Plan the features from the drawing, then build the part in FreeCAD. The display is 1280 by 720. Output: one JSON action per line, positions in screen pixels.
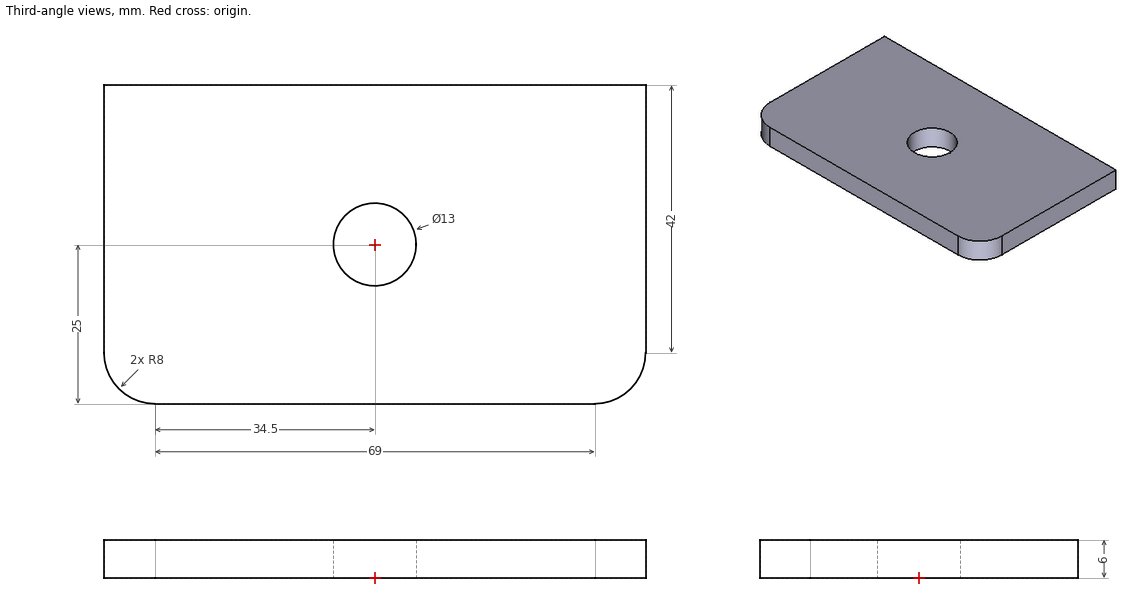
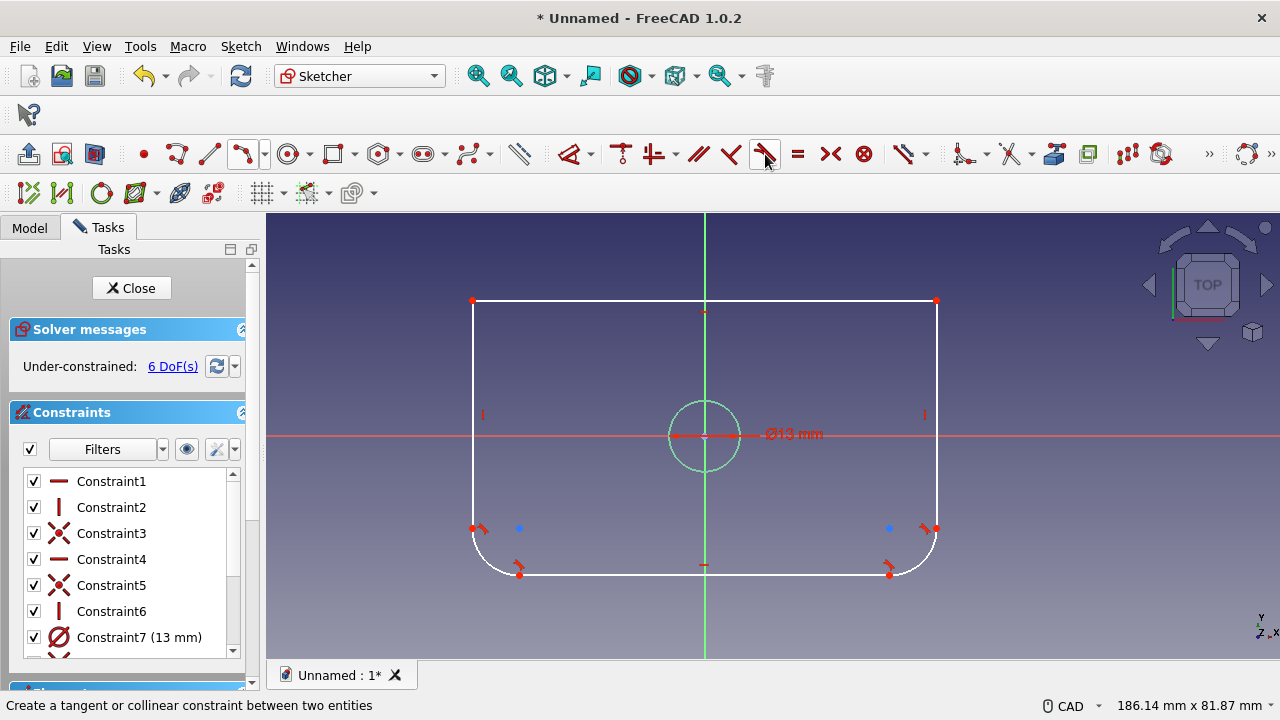
{"action": "left_click", "coordinate": [911, 570]}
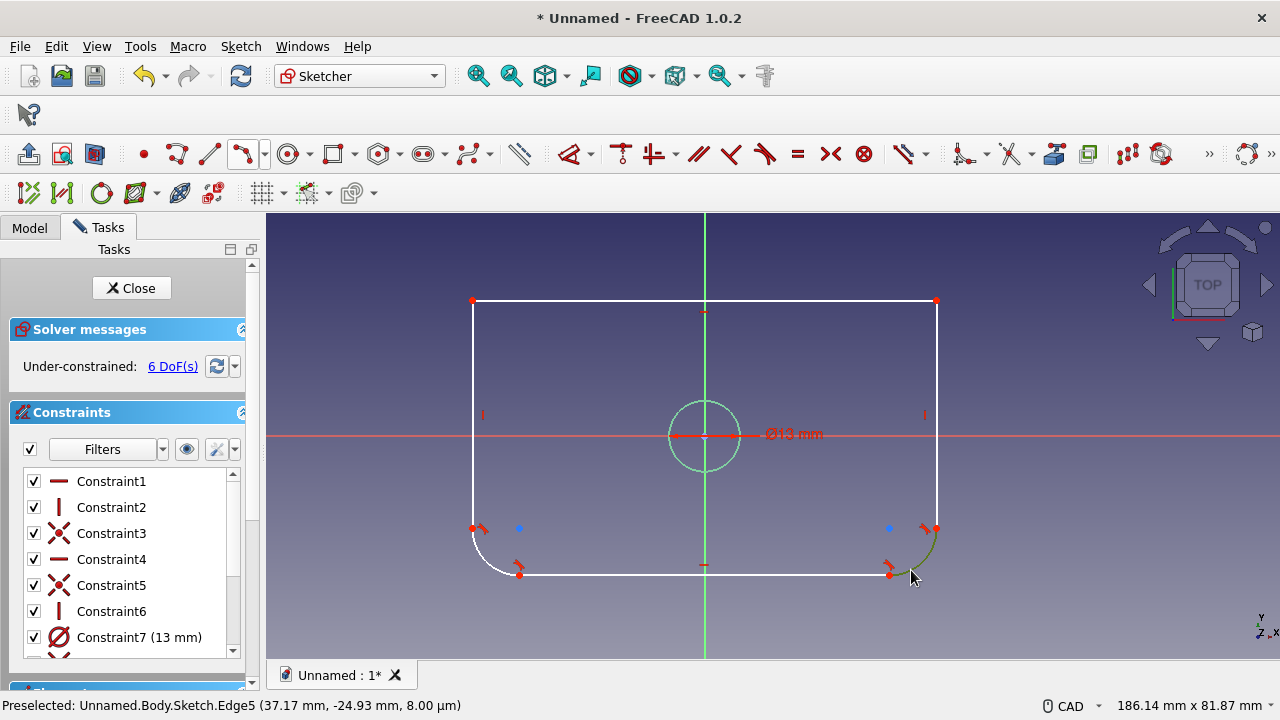
{"action": "left_click", "coordinate": [478, 550]}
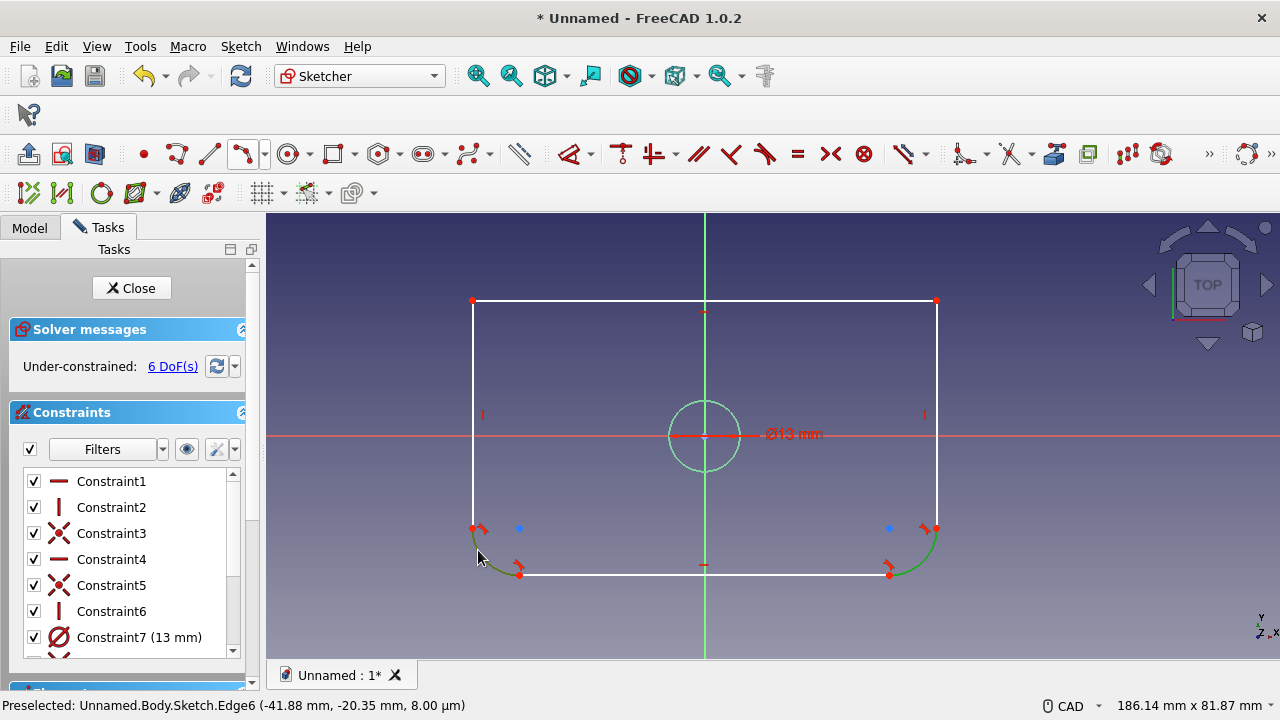
{"action": "left_click", "coordinate": [798, 154]}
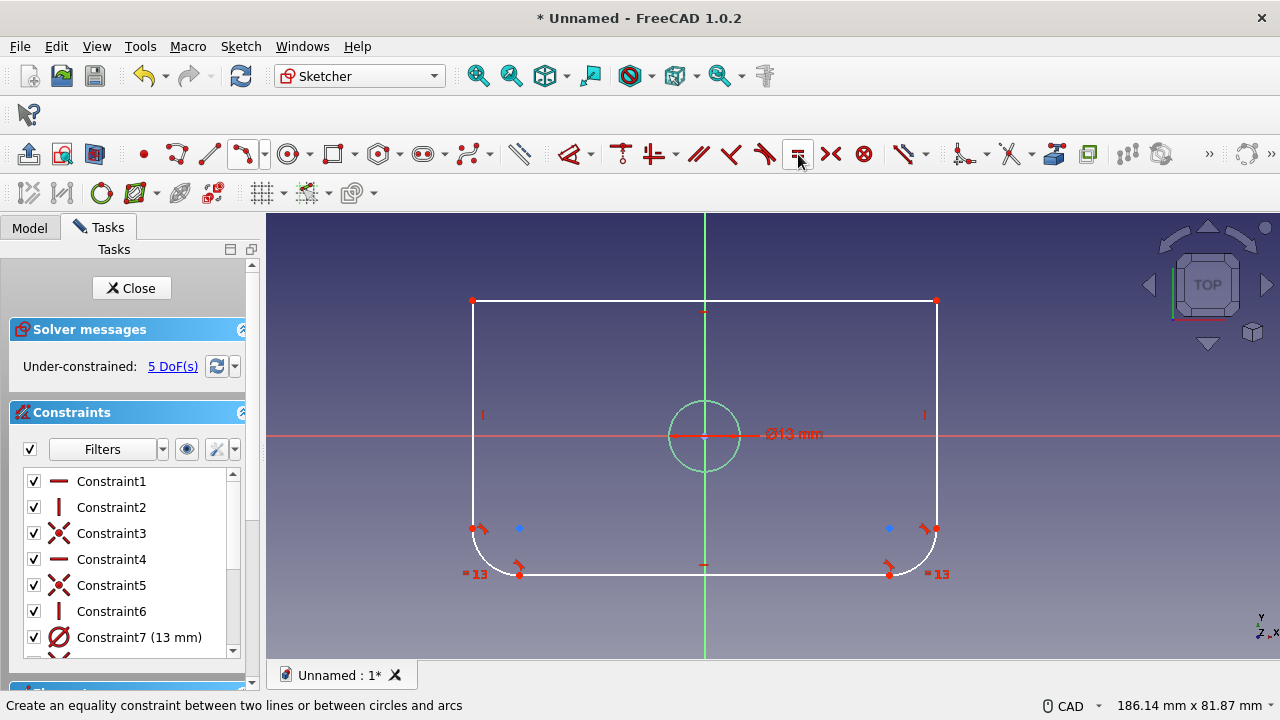
{"action": "left_click", "coordinate": [568, 154]}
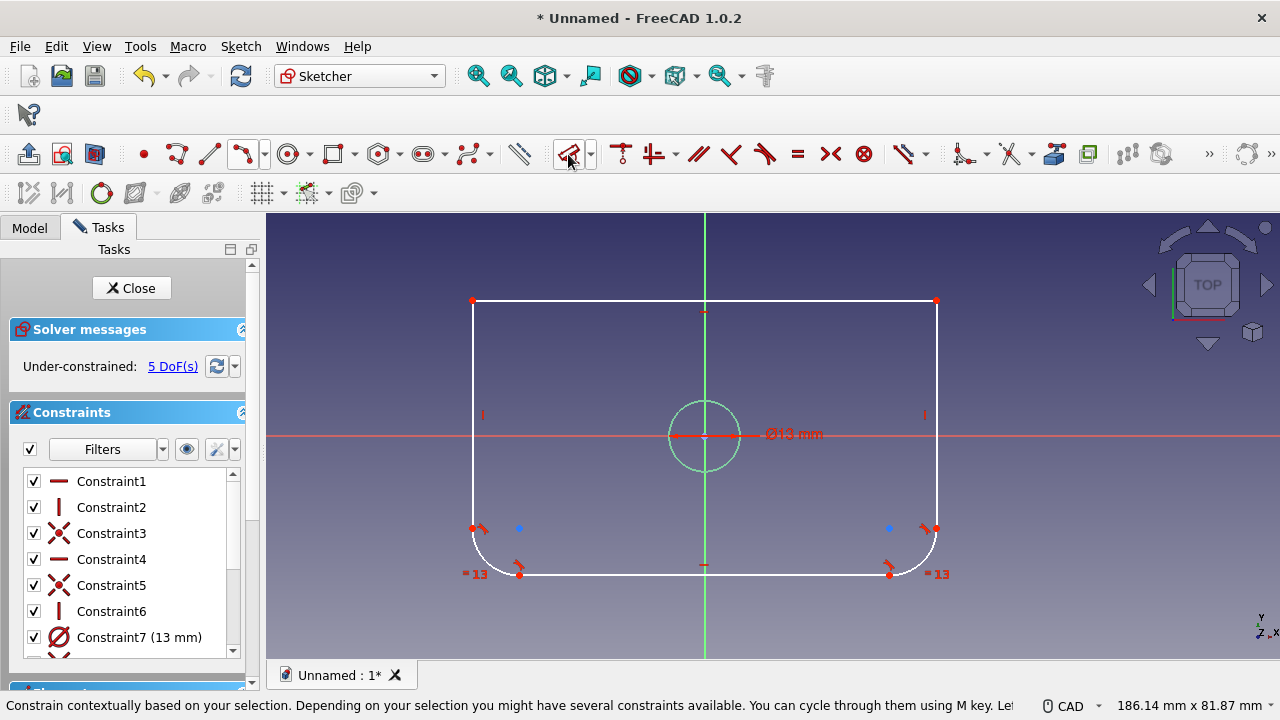
{"action": "left_click", "coordinate": [911, 570]}
{"action": "left_click", "coordinate": [926, 598]}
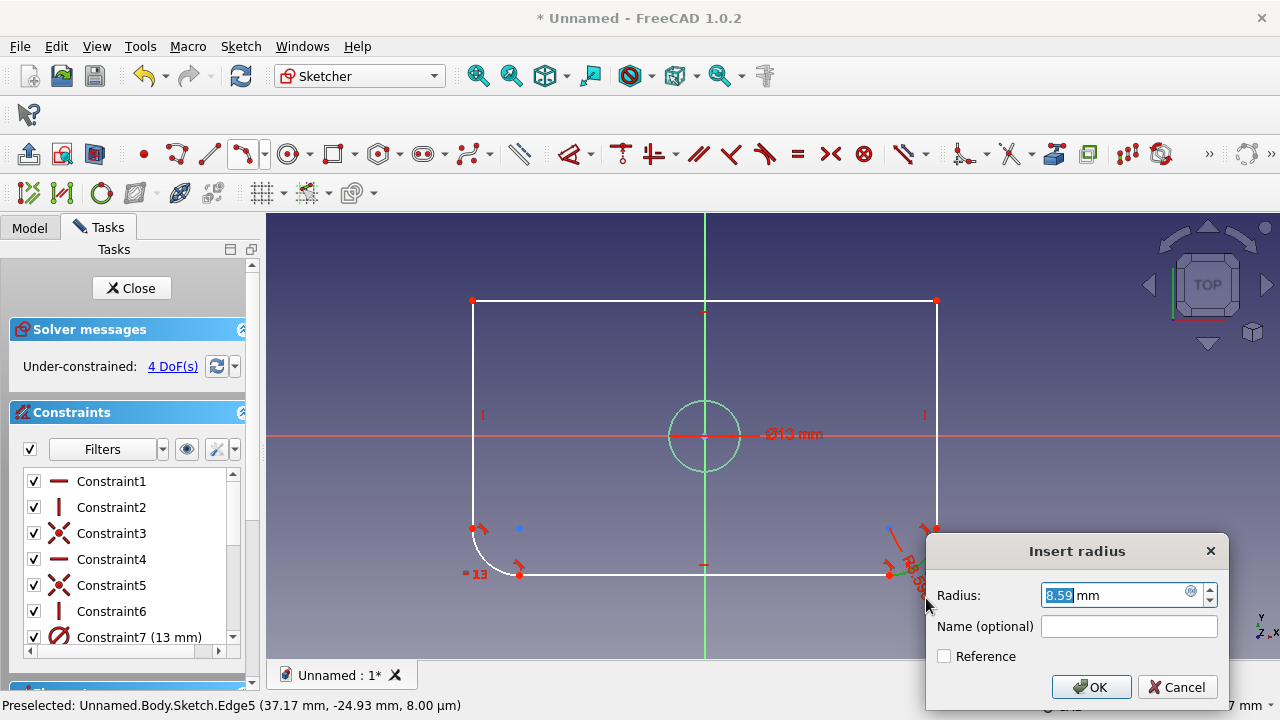
{"action": "type", "text": "8"}
{"action": "key", "text": "Return"}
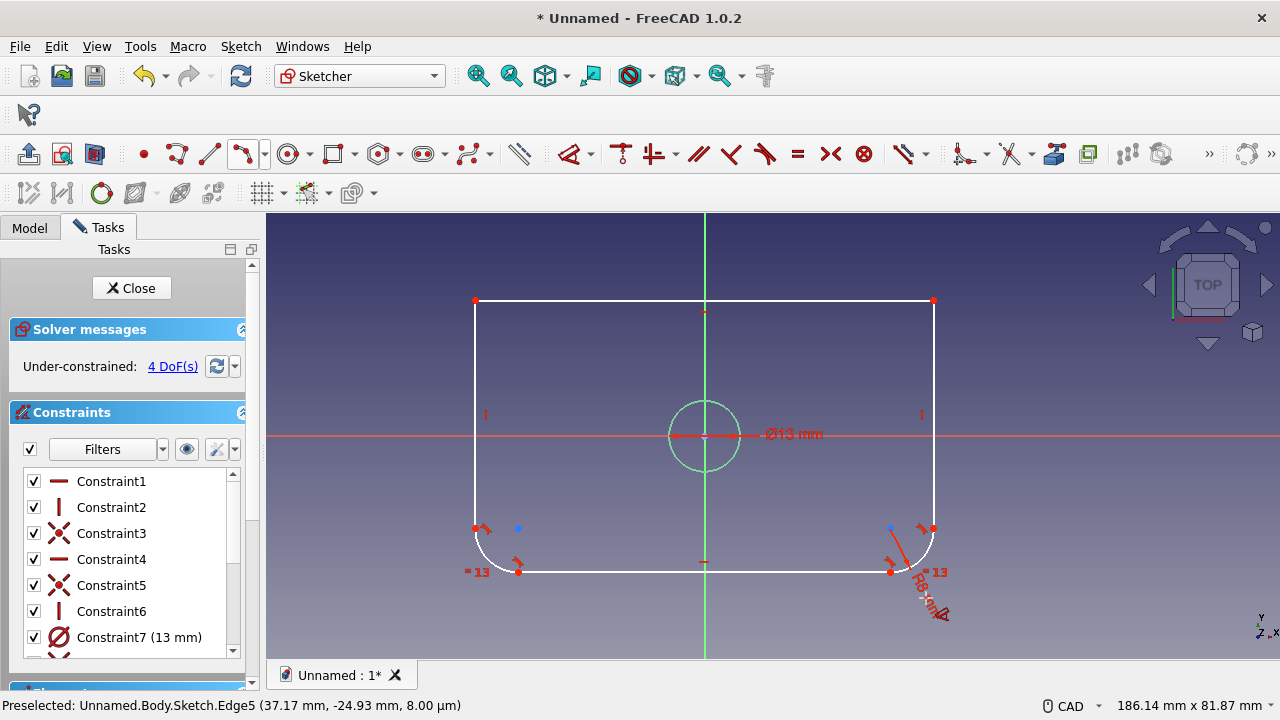
{"action": "left_click", "coordinate": [630, 572]}
{"action": "left_click", "coordinate": [619, 606]}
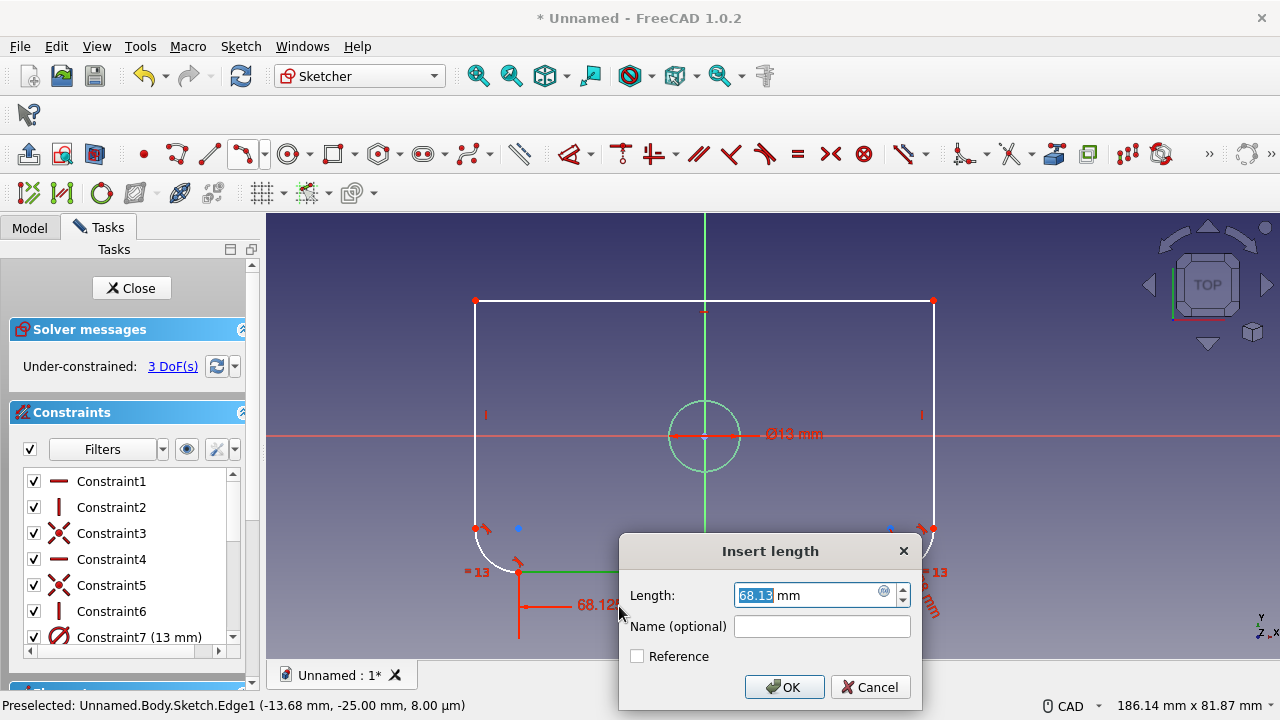
{"action": "type", "text": "69"}
{"action": "key", "text": "Return"}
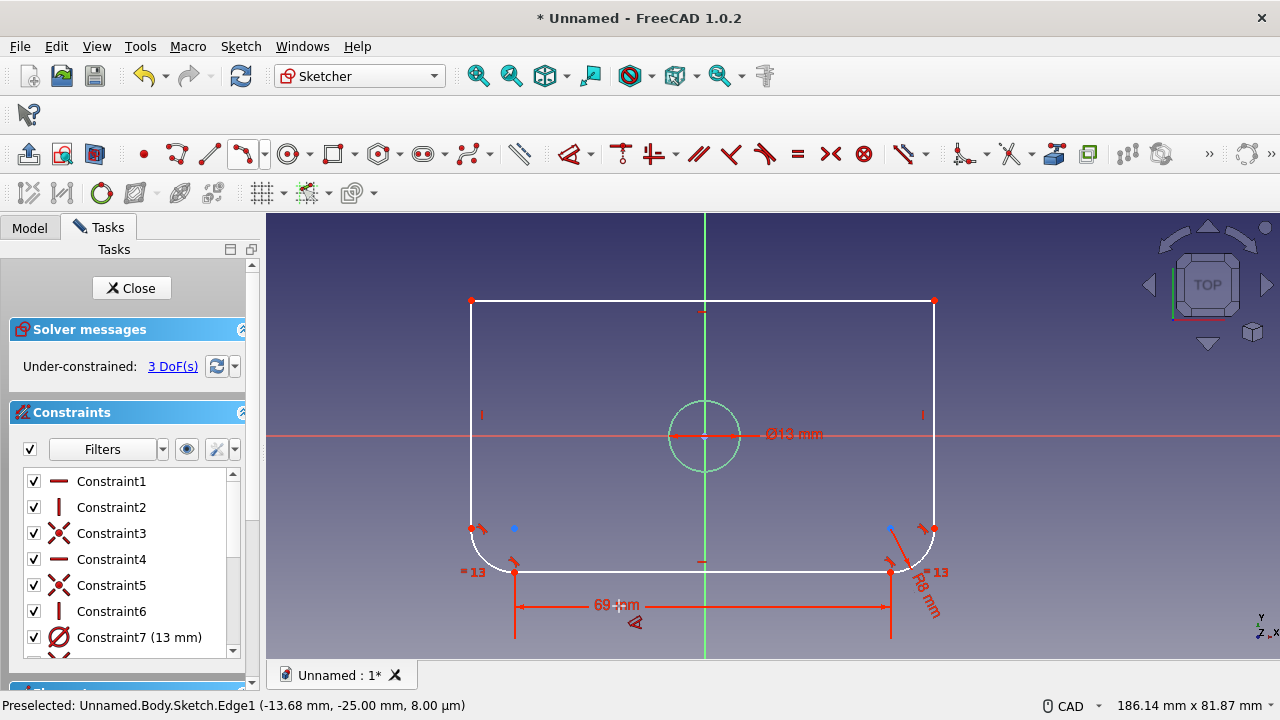
{"action": "left_click", "coordinate": [934, 460]}
{"action": "left_click", "coordinate": [968, 415]}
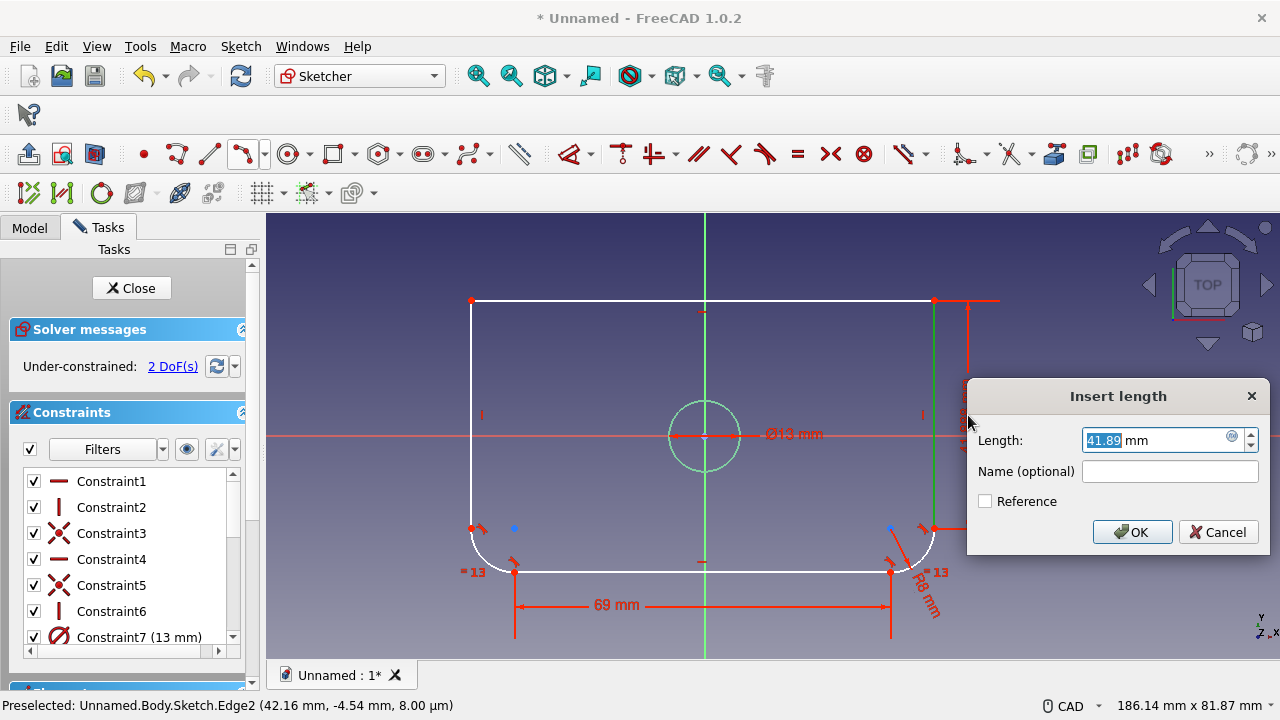
{"action": "type", "text": "42"}
{"action": "key", "text": "Return"}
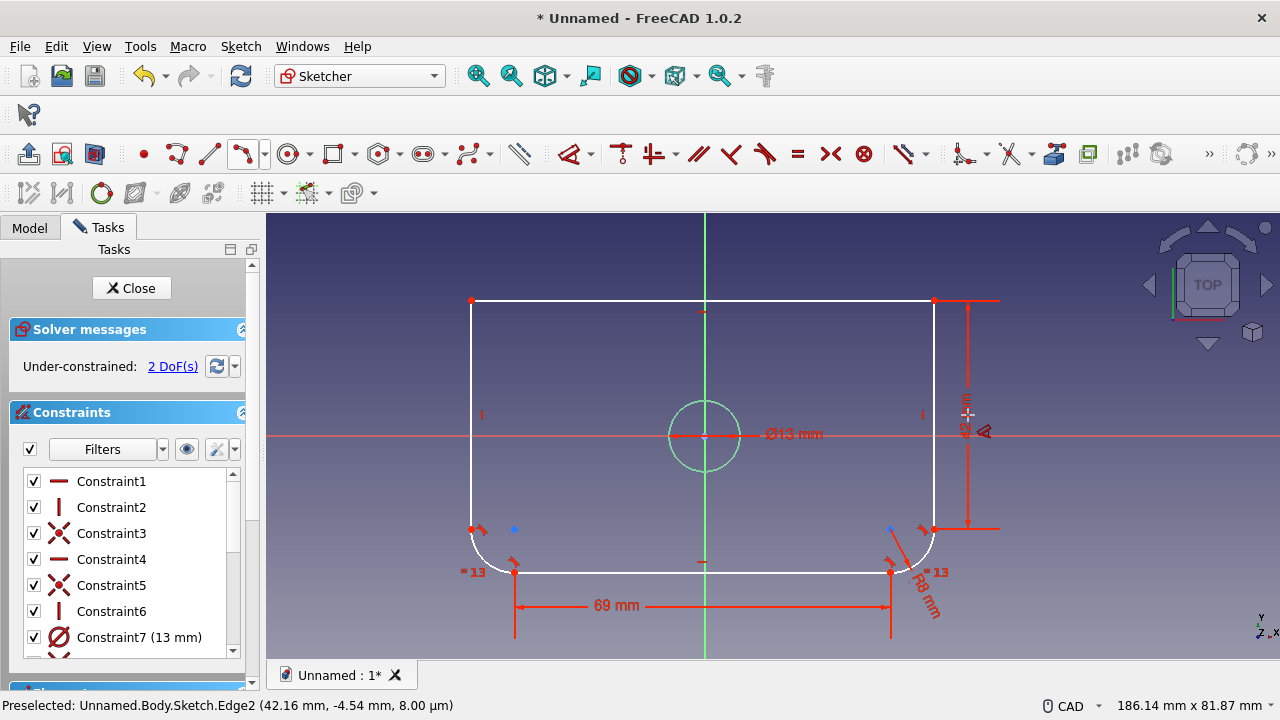
{"action": "left_click", "coordinate": [515, 573]}
{"action": "left_click", "coordinate": [739, 505]}